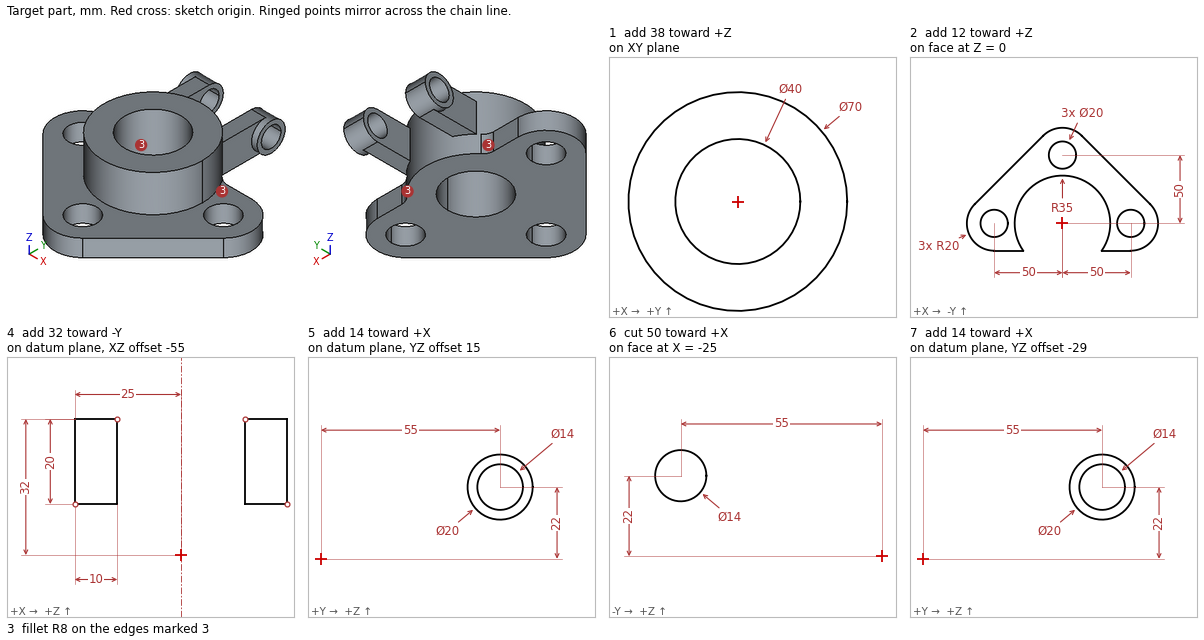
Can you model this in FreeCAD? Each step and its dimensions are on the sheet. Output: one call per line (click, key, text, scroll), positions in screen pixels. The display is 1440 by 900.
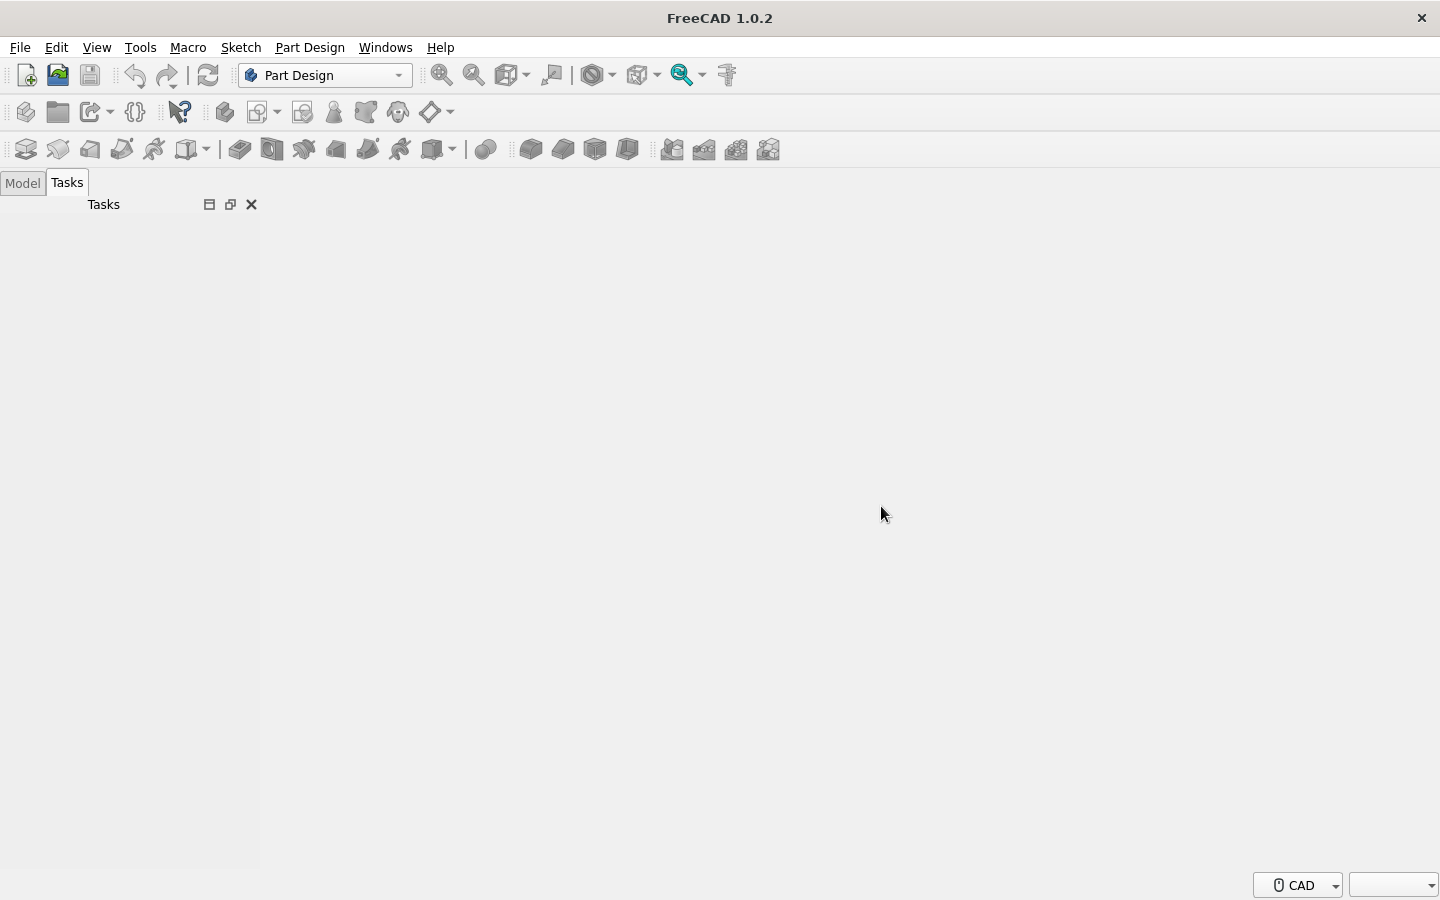
key(ctrl+n)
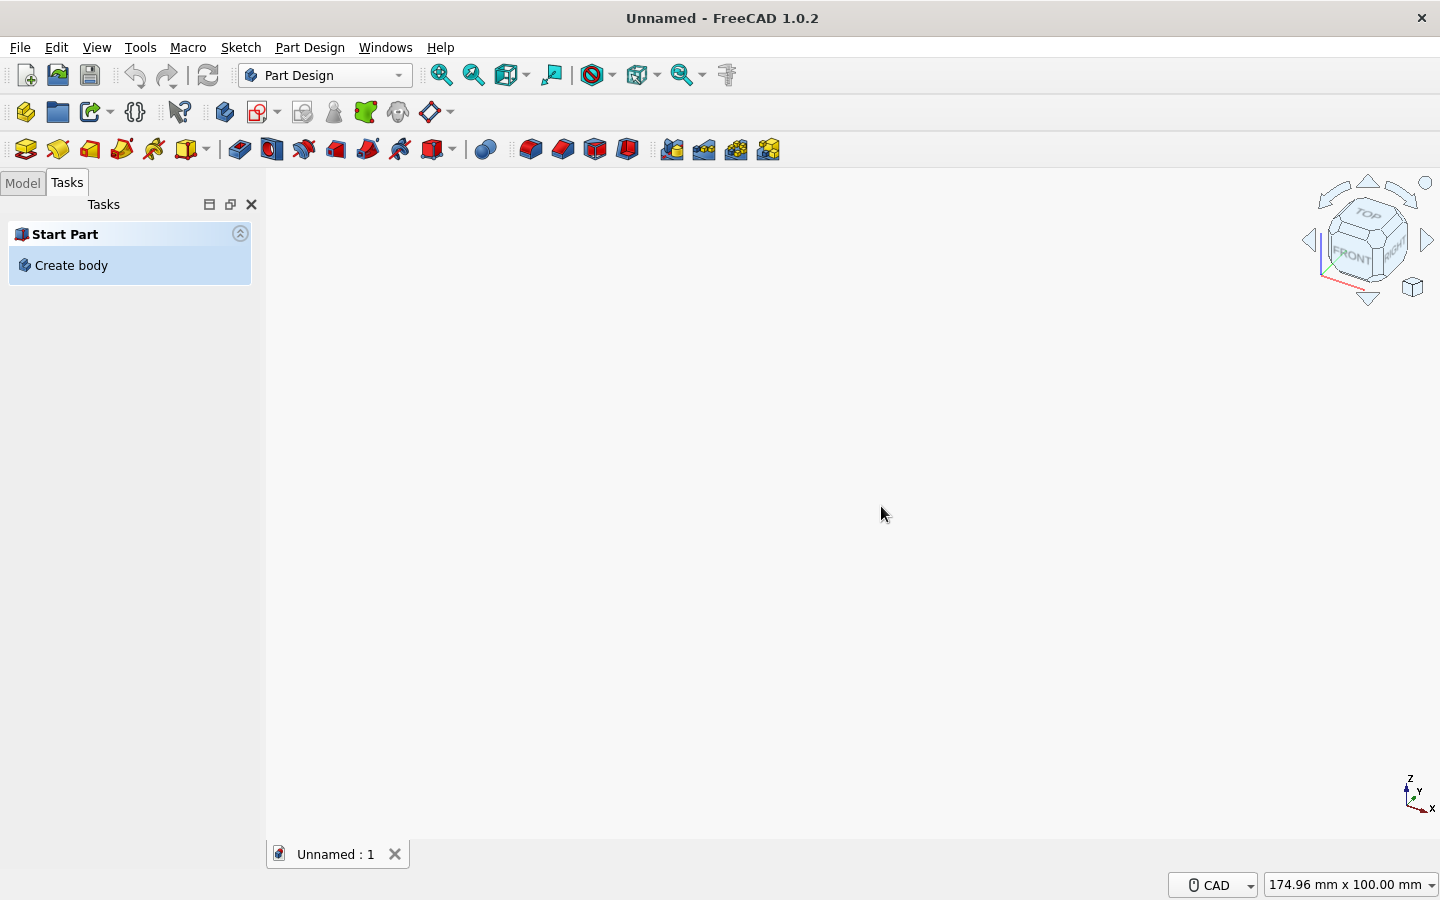
click(258, 112)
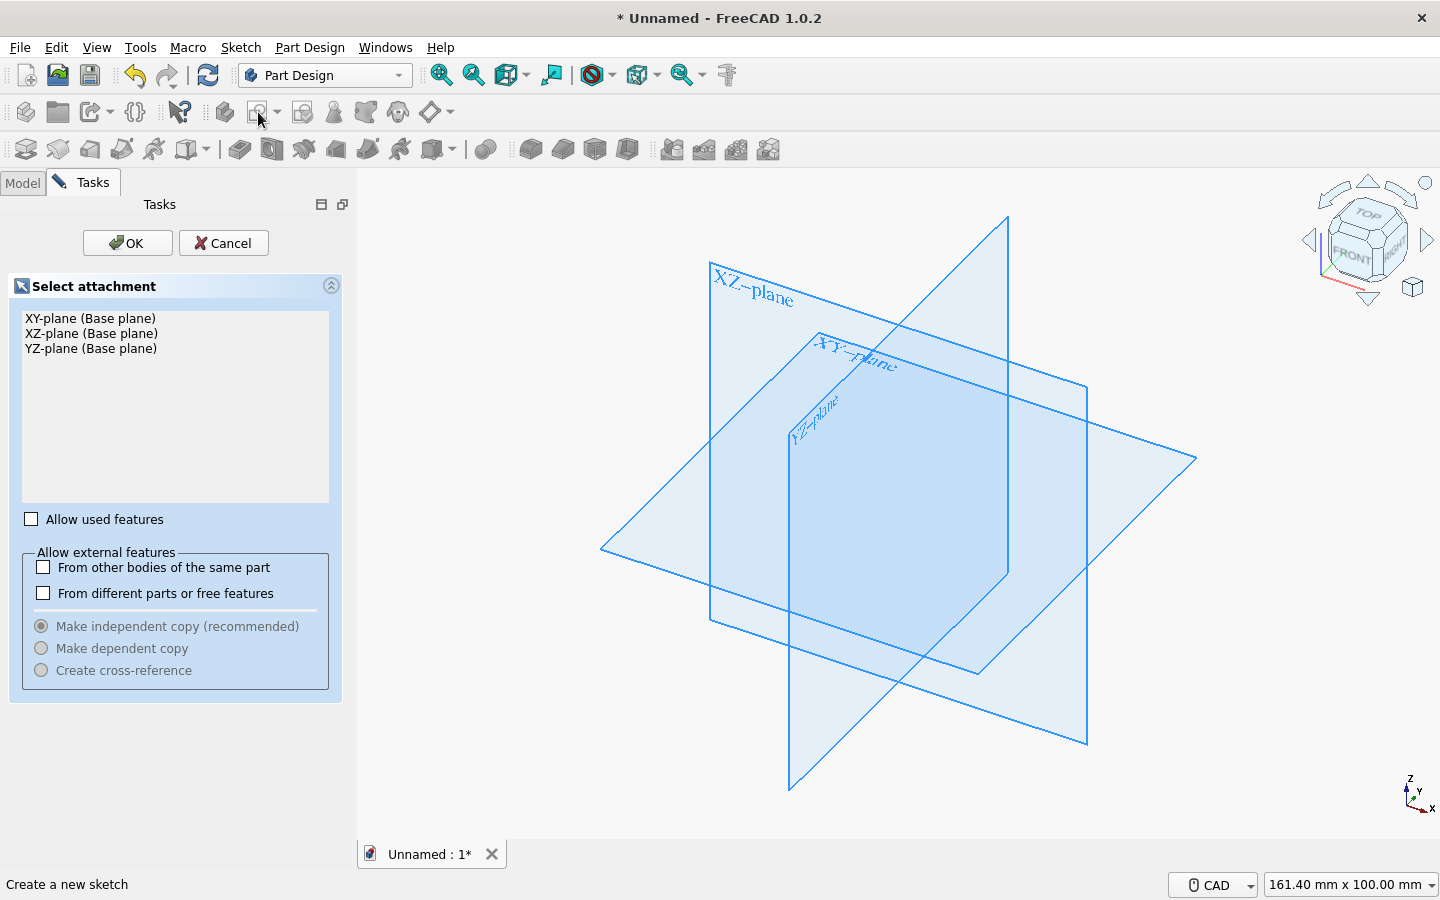
click(82, 318)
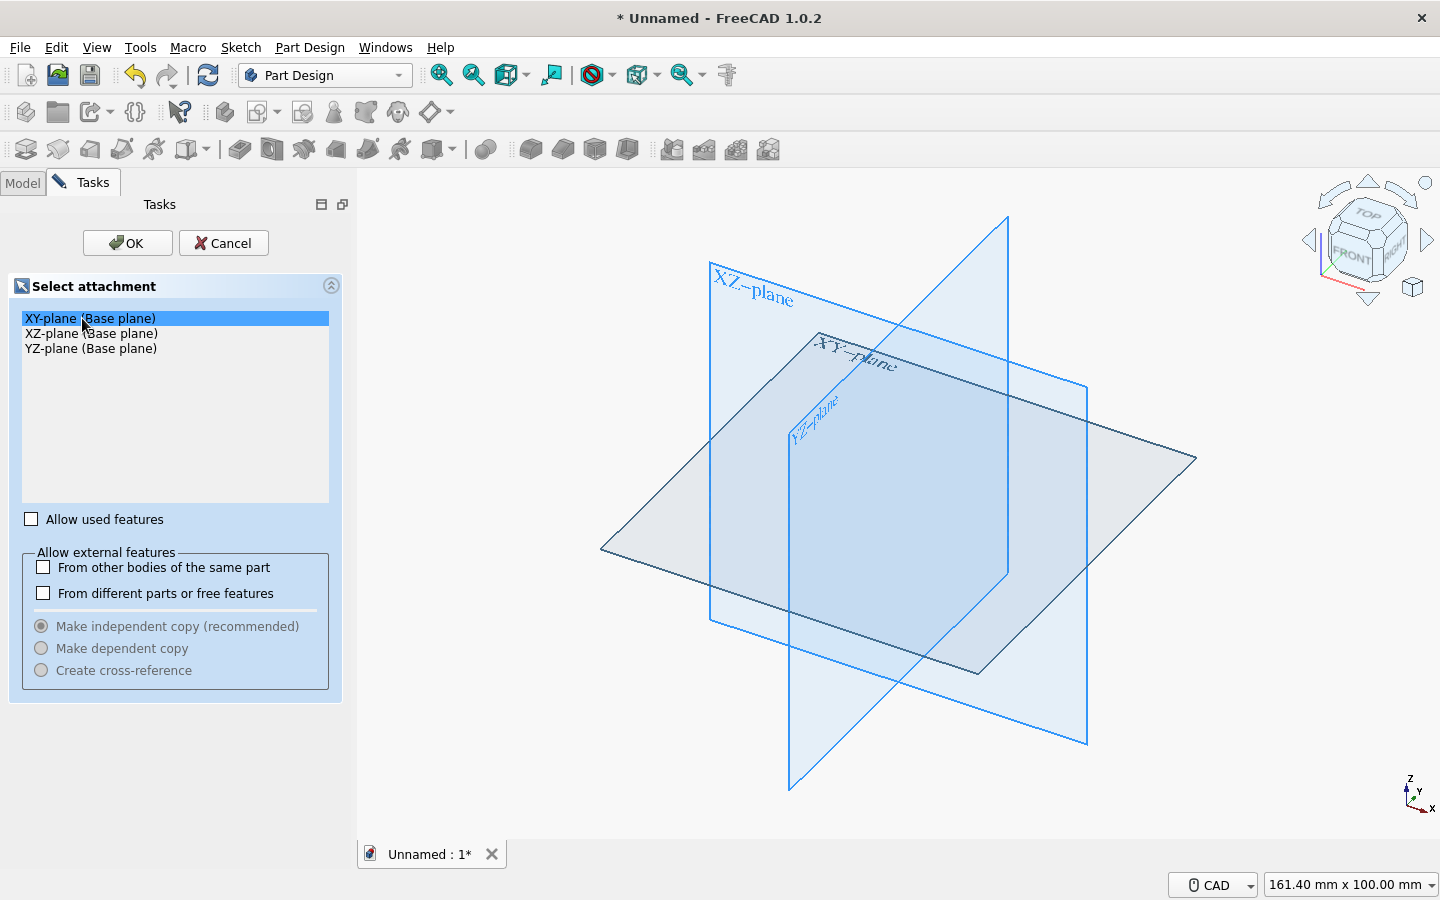
click(128, 243)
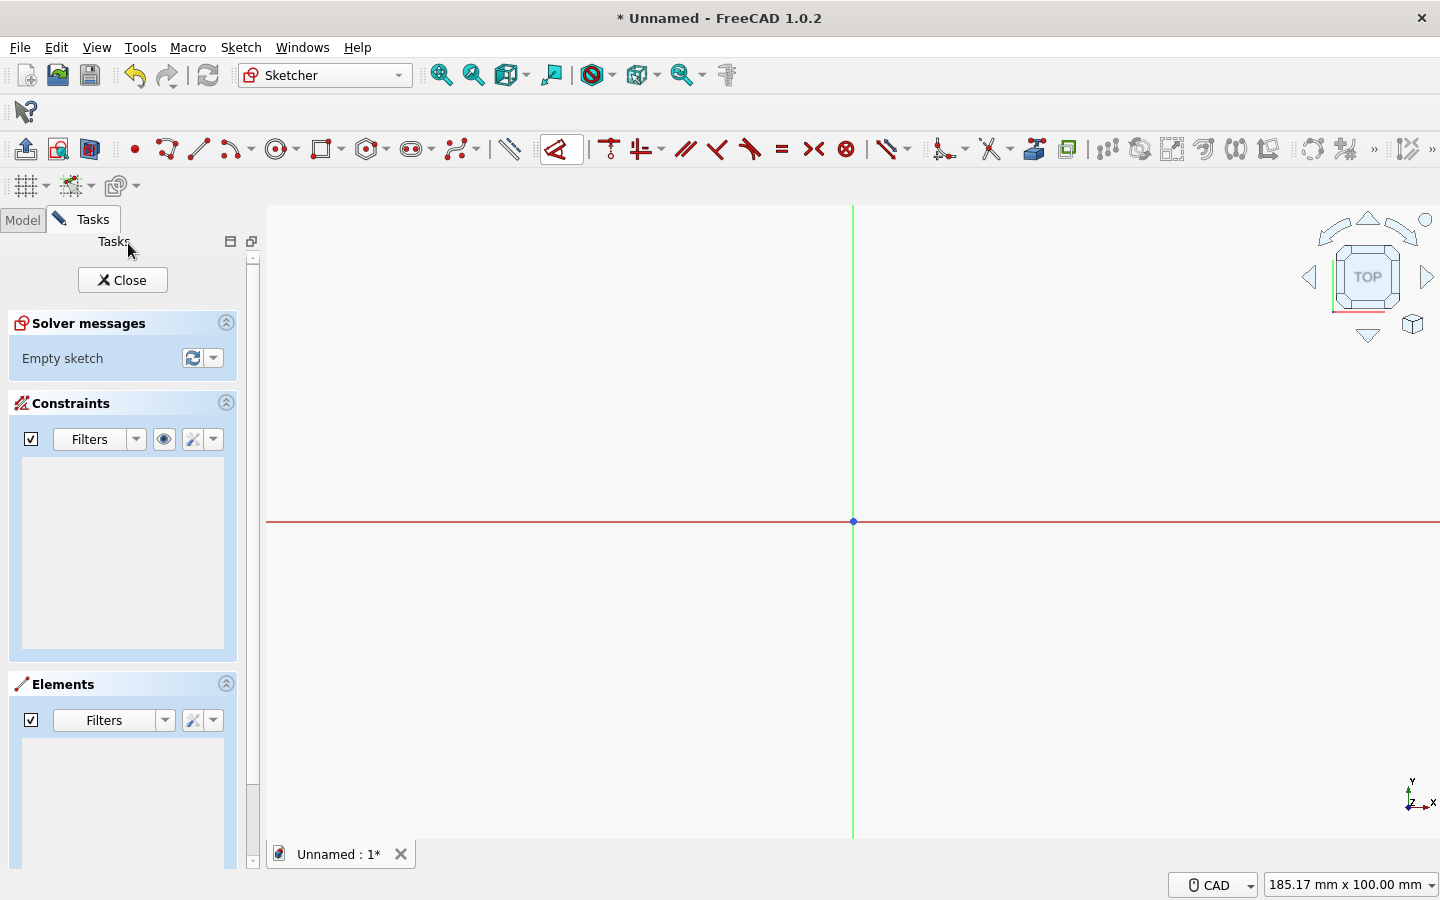
key(g)
key(c)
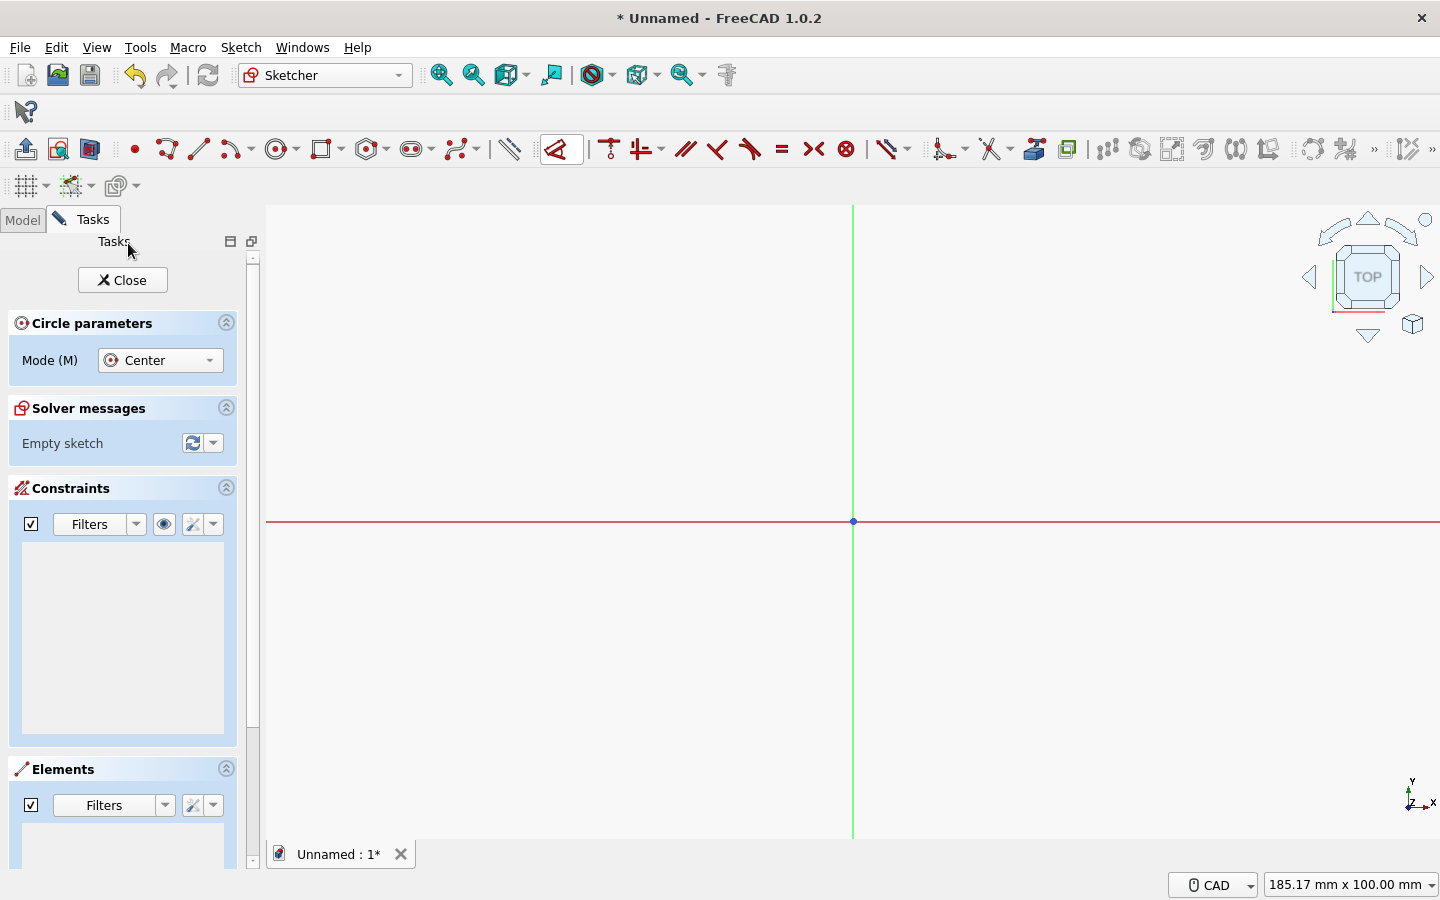
click(853, 522)
click(1010, 365)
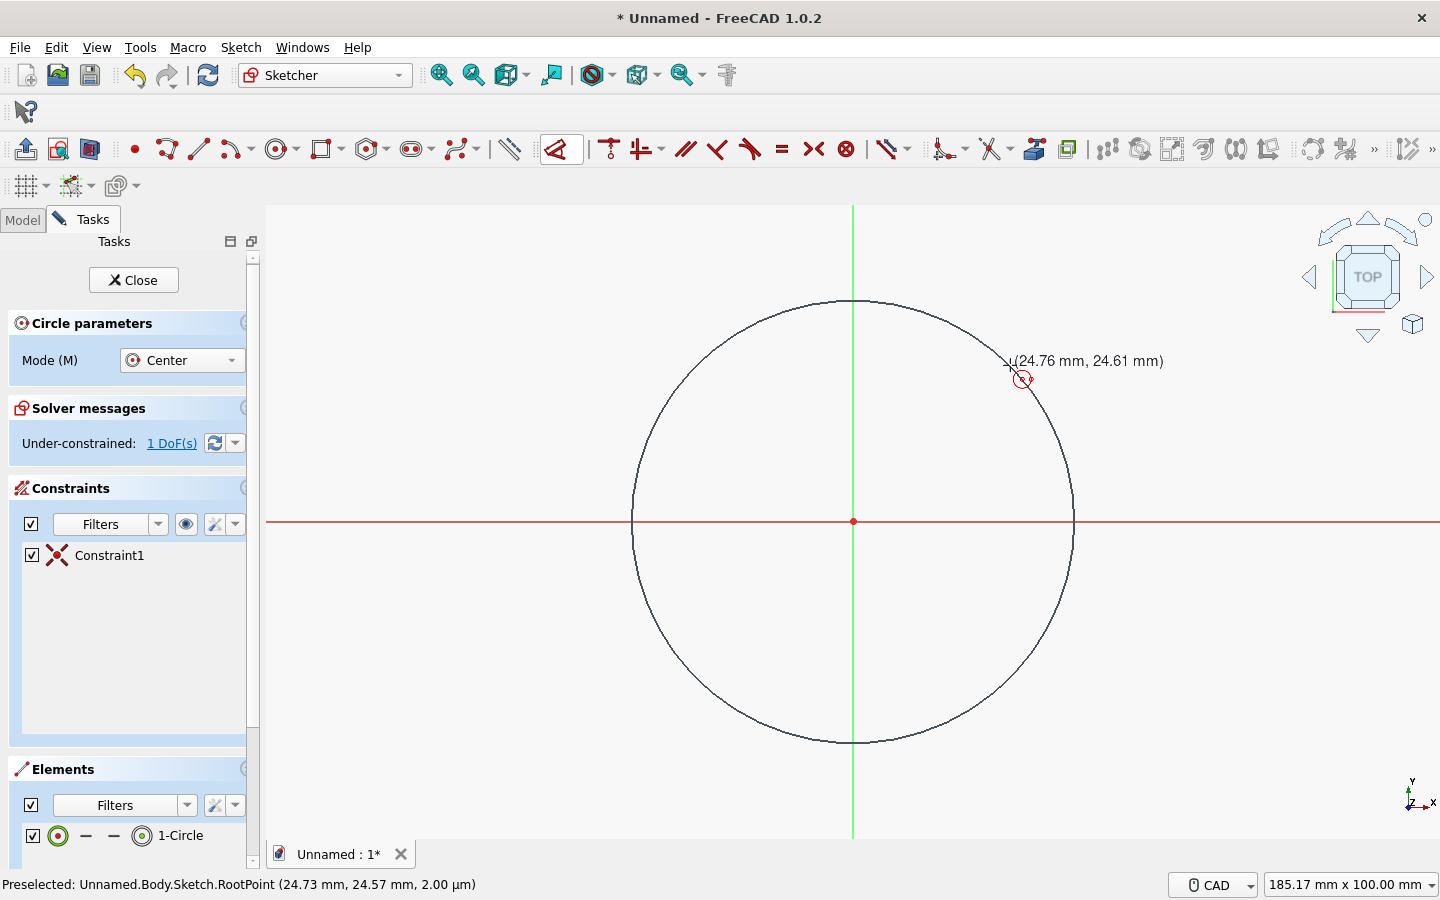
click(853, 522)
click(943, 432)
key(Escape)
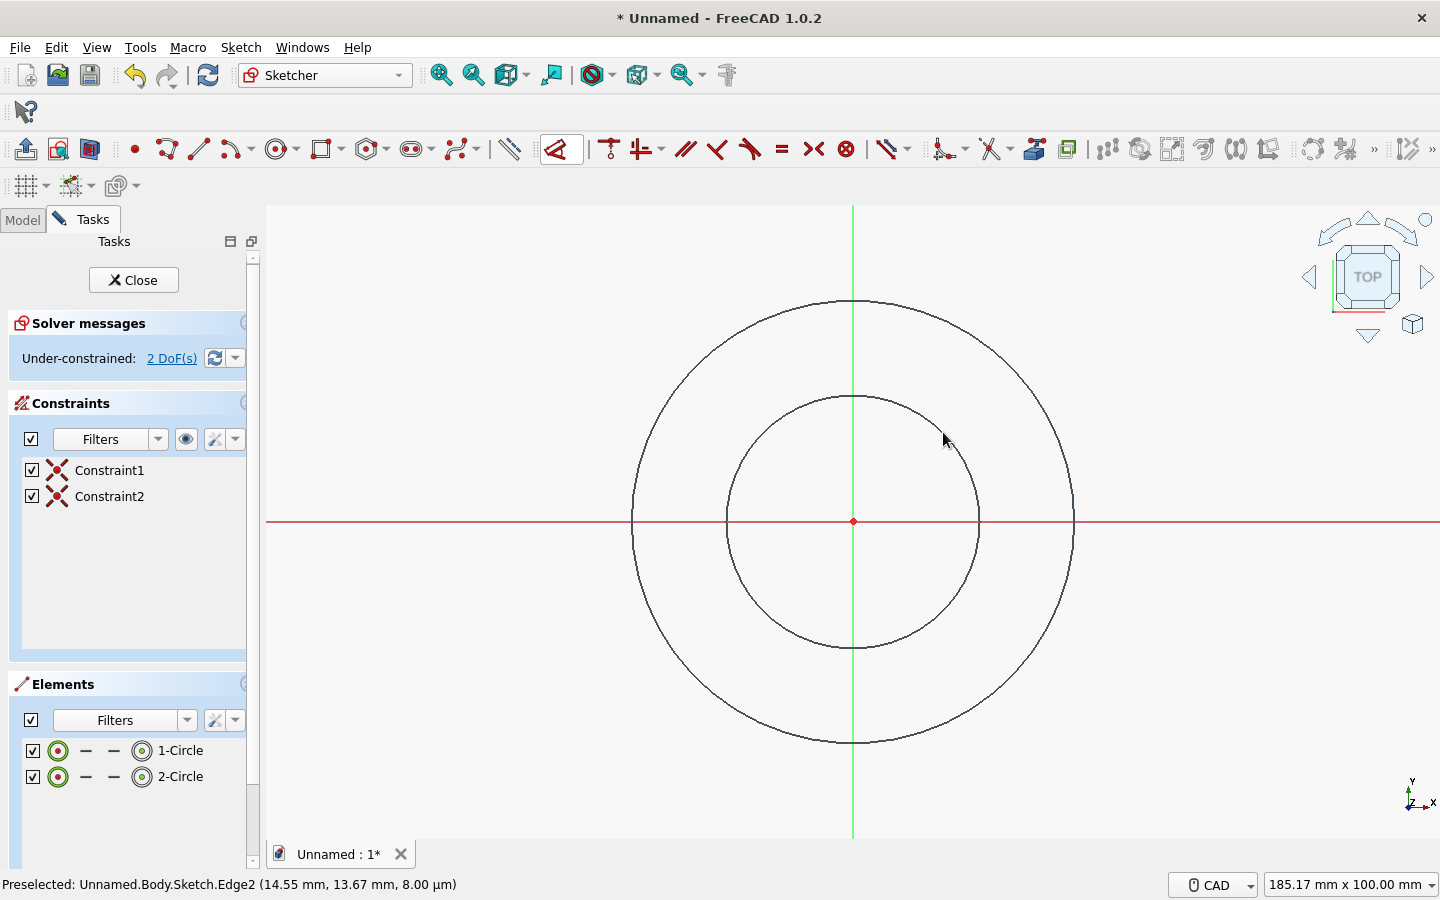
click(556, 150)